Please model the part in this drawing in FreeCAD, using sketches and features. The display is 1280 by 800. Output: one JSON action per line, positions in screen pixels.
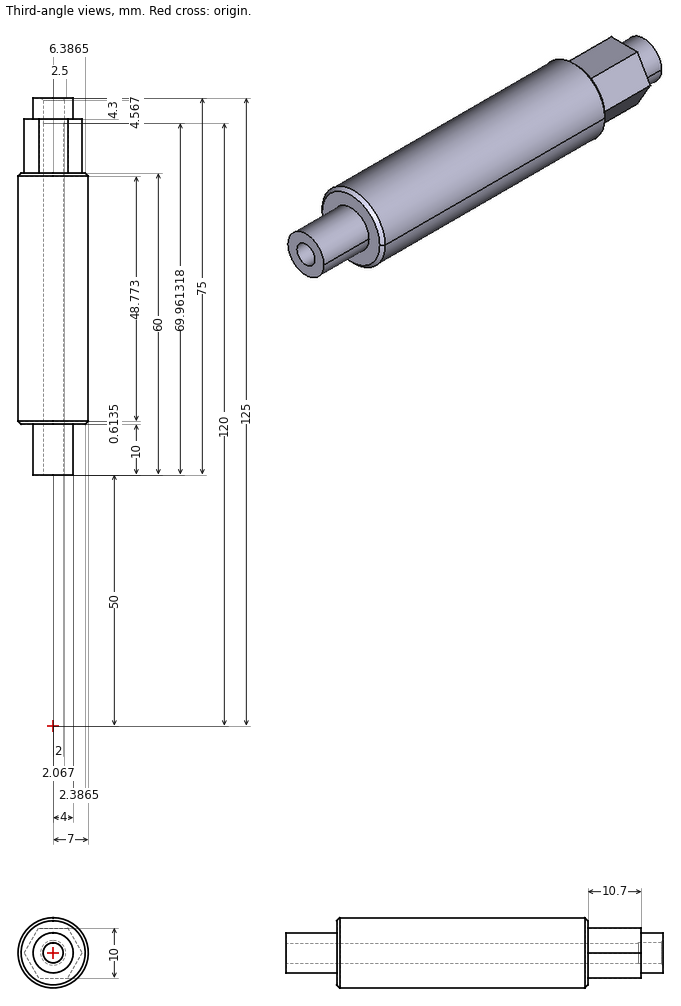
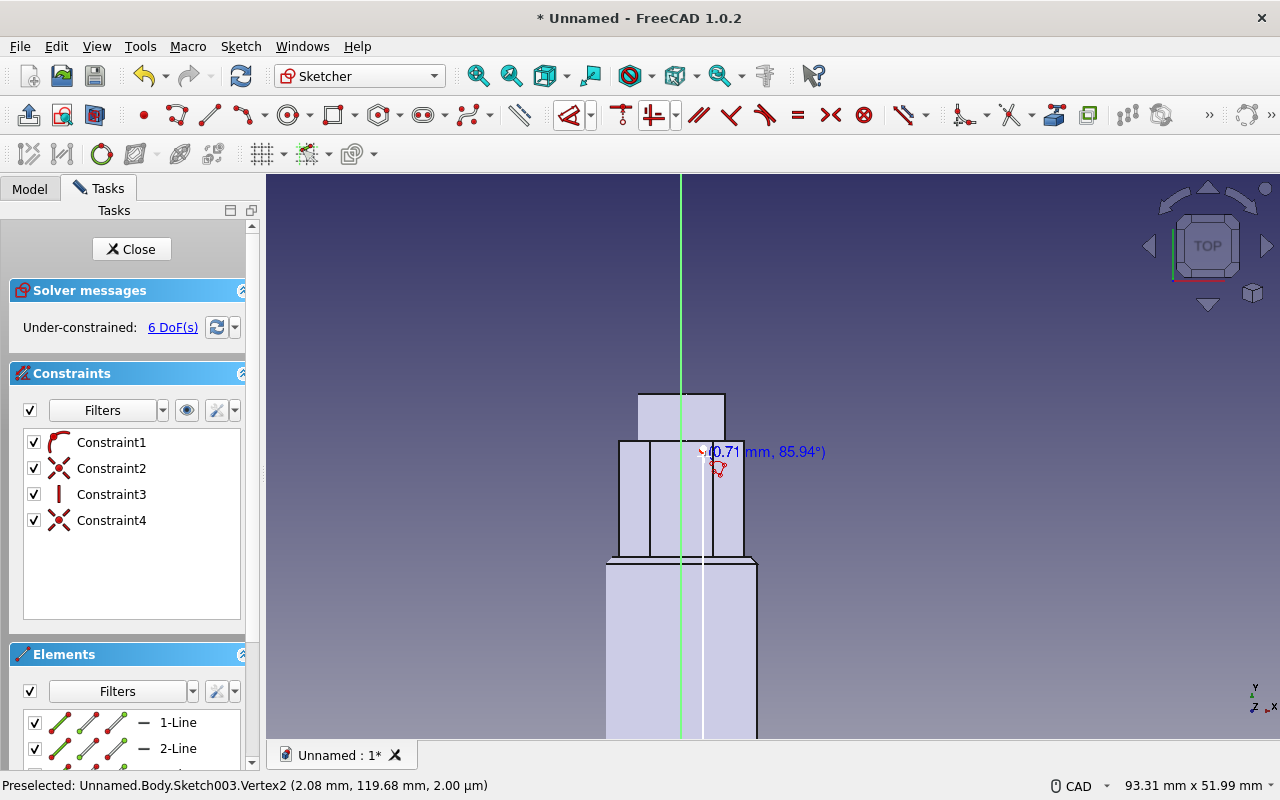
{"action": "scroll", "coordinate": [708, 255], "scroll_direction": "down", "scroll_amount": 7}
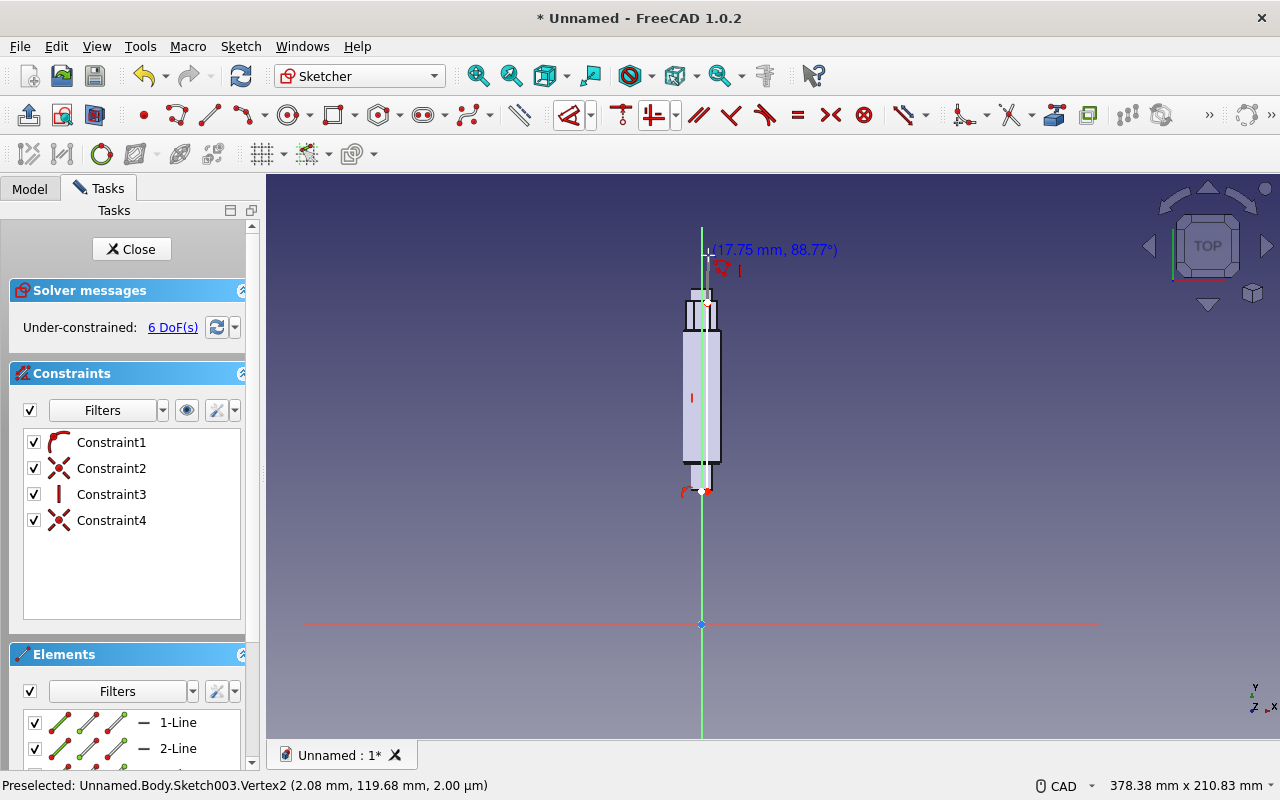
{"action": "scroll", "coordinate": [707, 291], "scroll_direction": "up", "scroll_amount": 6}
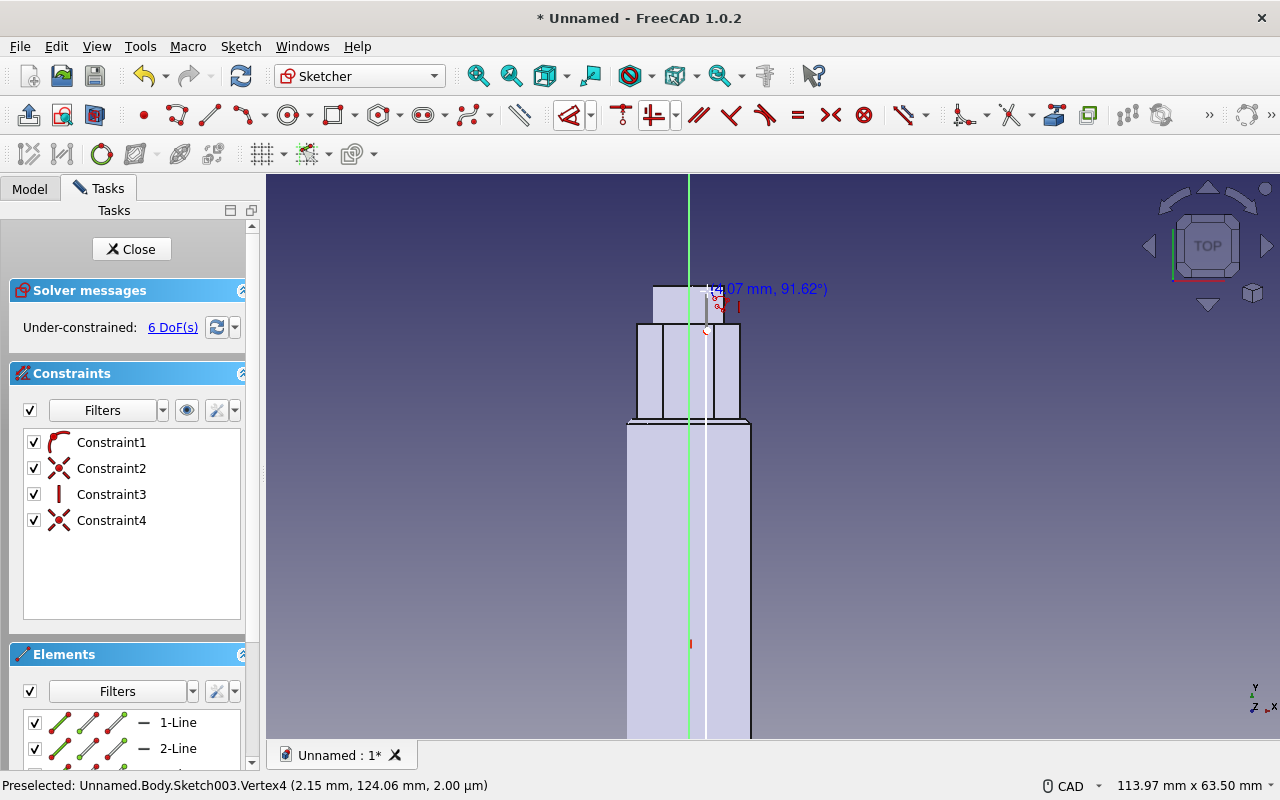
{"action": "left_click", "coordinate": [707, 289]}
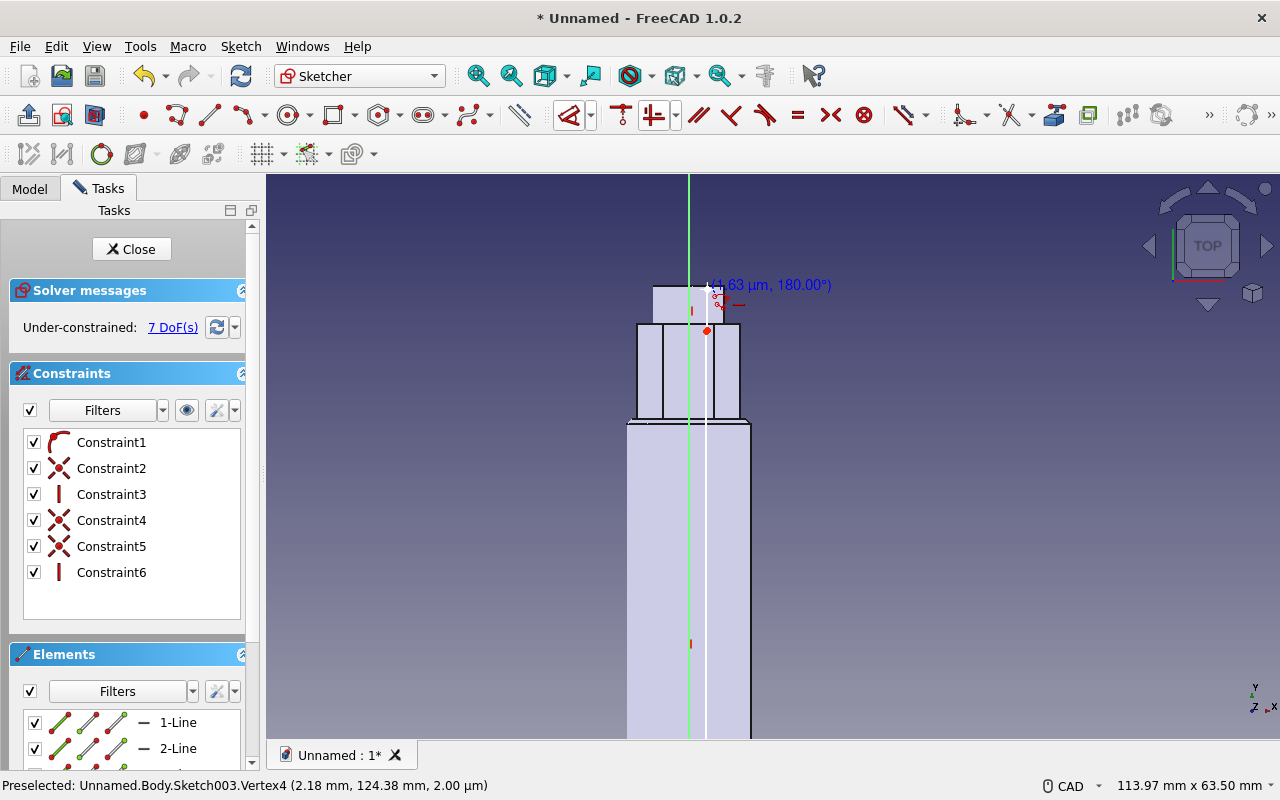
{"action": "scroll", "coordinate": [711, 286], "scroll_direction": "up", "scroll_amount": 6}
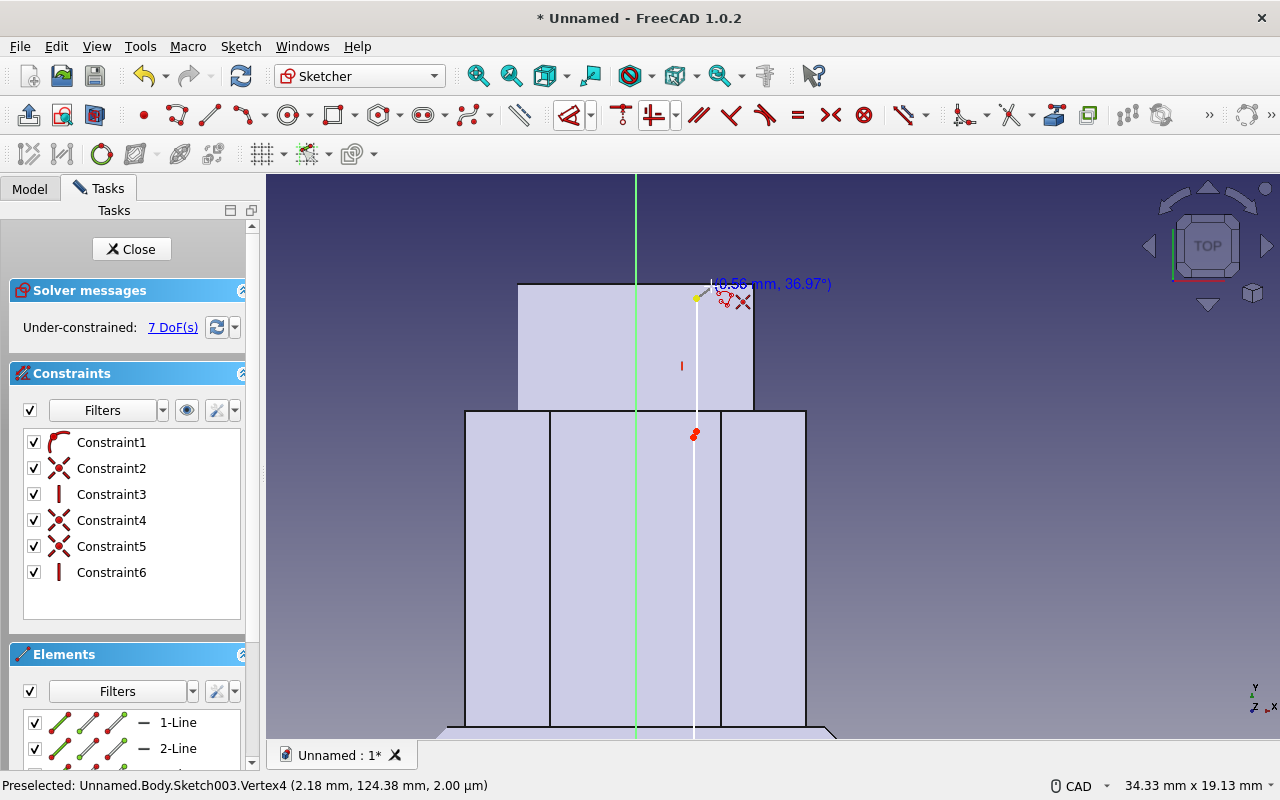
{"action": "left_click", "coordinate": [710, 284]}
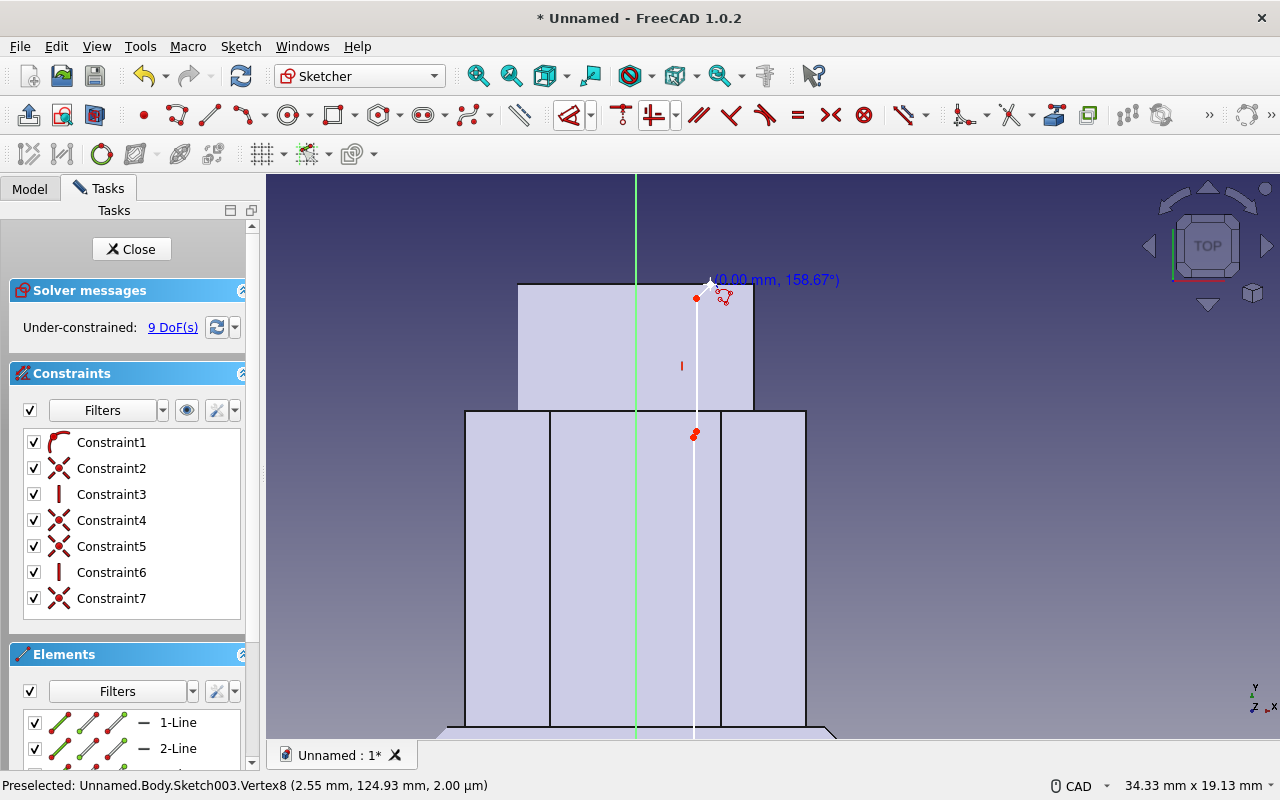
{"action": "scroll", "coordinate": [708, 290], "scroll_direction": "down", "scroll_amount": 12}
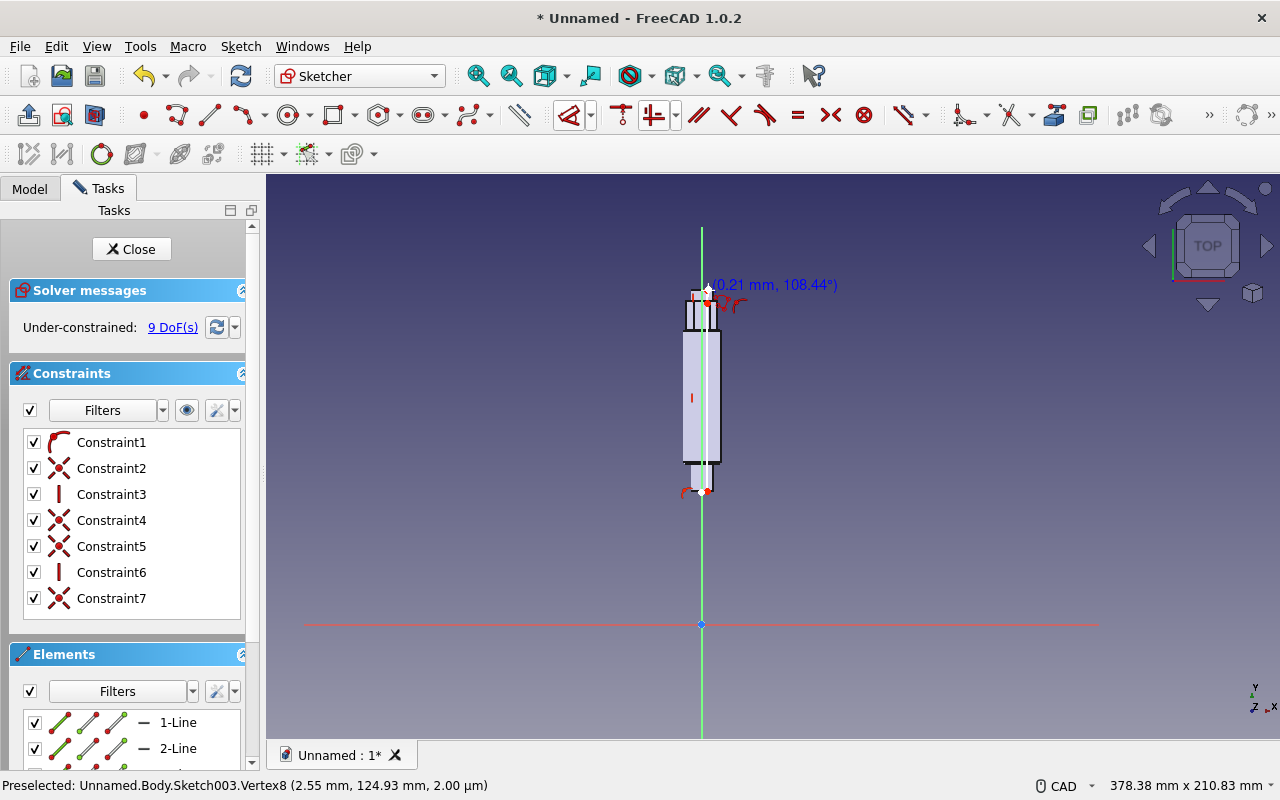
{"action": "scroll", "coordinate": [702, 290], "scroll_direction": "up", "scroll_amount": 6}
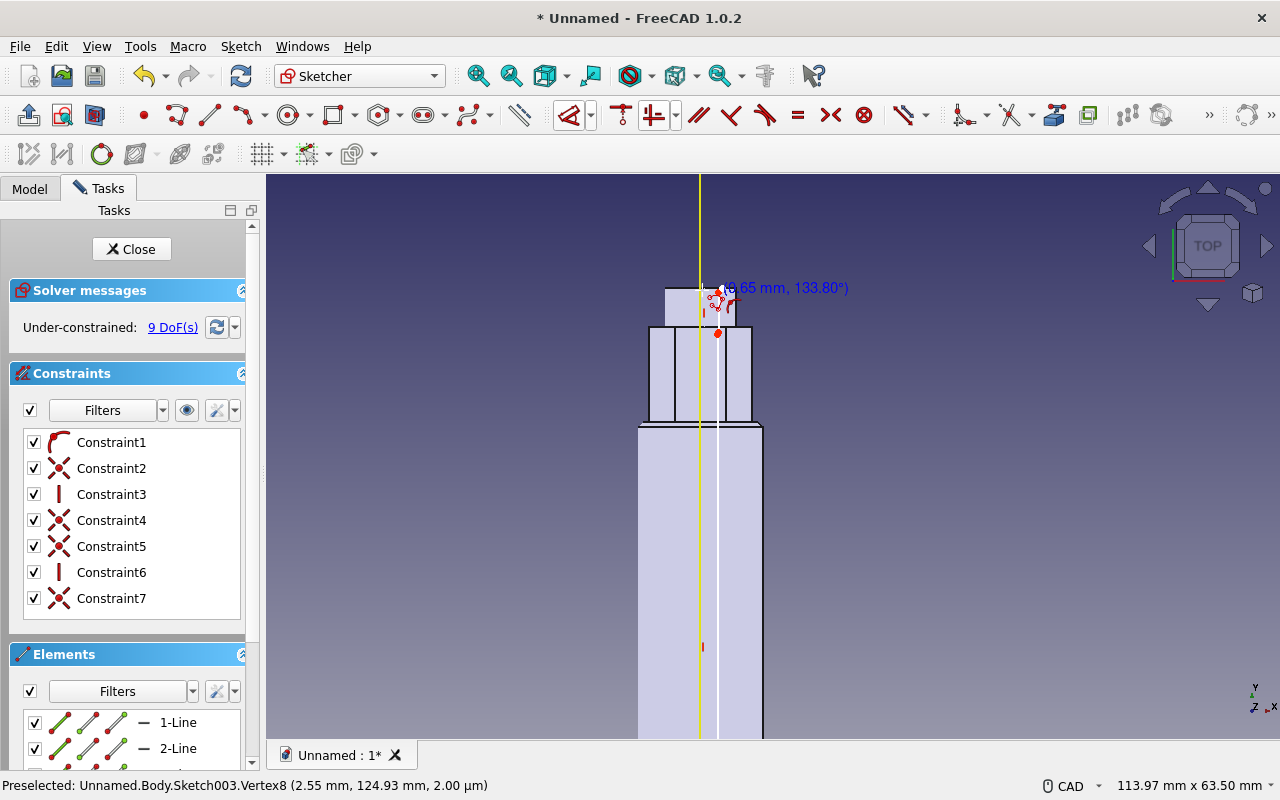
{"action": "left_click", "coordinate": [709, 288]}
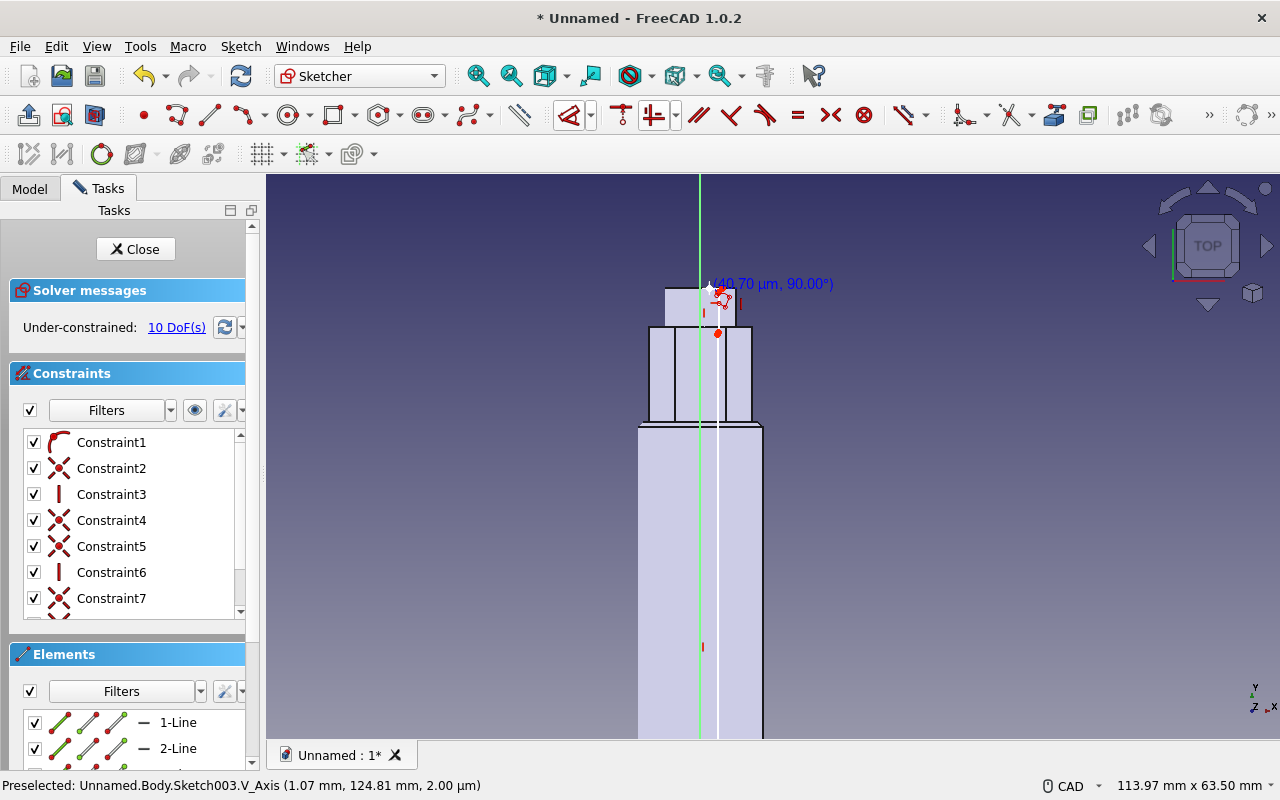
{"action": "scroll", "coordinate": [701, 289], "scroll_direction": "down", "scroll_amount": 6}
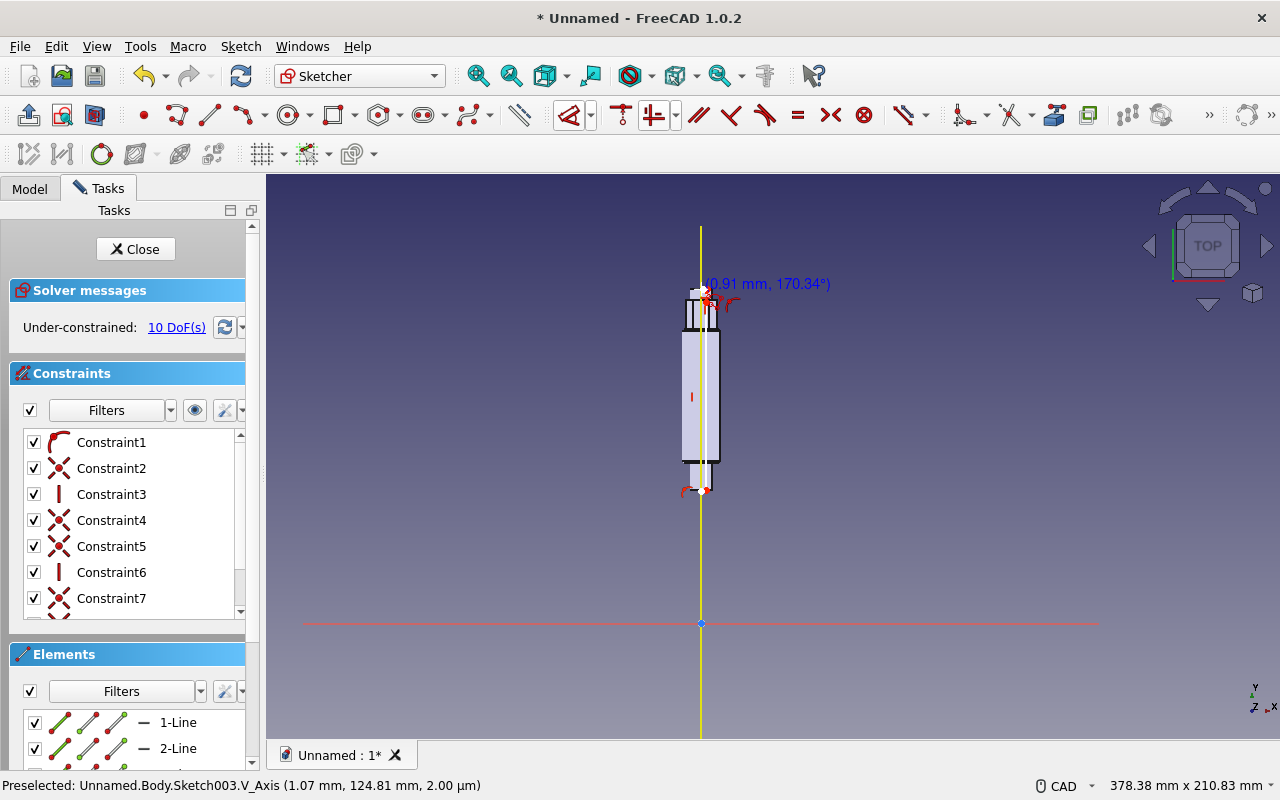
{"action": "scroll", "coordinate": [701, 490], "scroll_direction": "up", "scroll_amount": 9}